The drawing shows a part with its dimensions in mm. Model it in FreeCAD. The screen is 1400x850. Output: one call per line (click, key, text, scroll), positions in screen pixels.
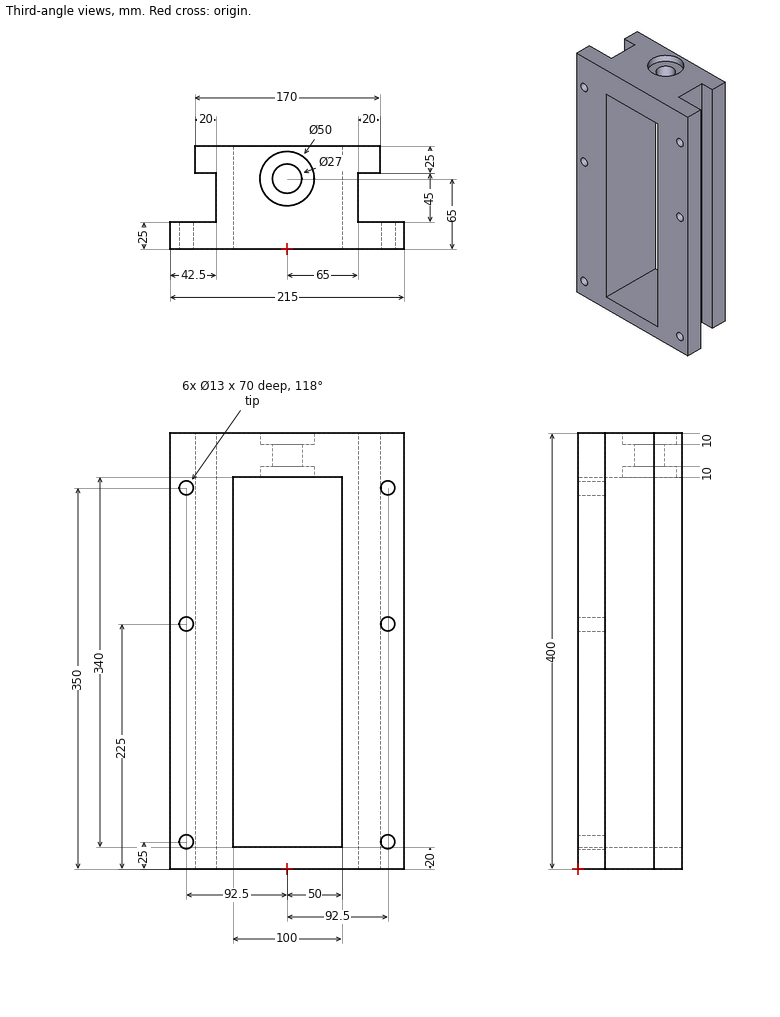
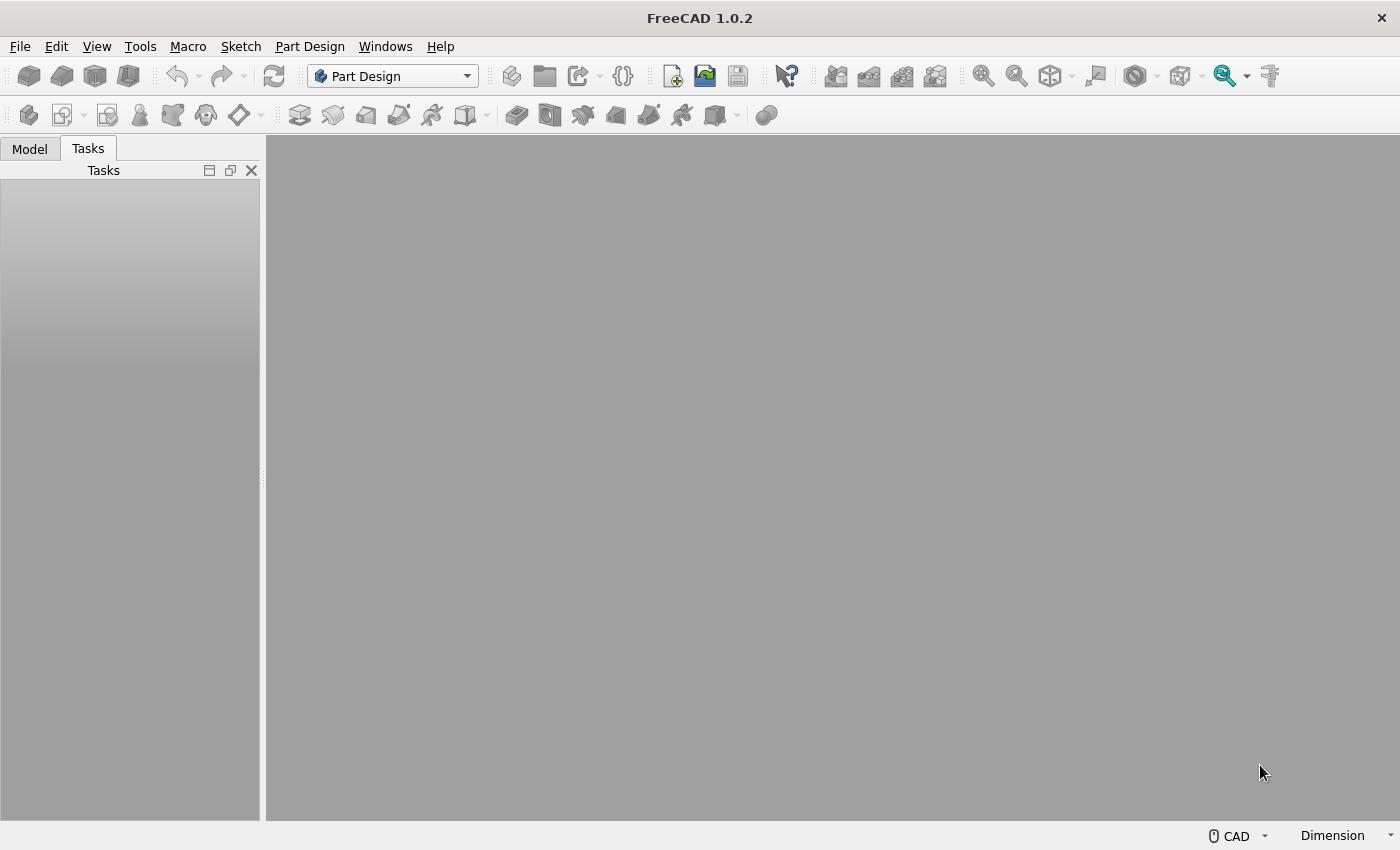
key(ctrl+n)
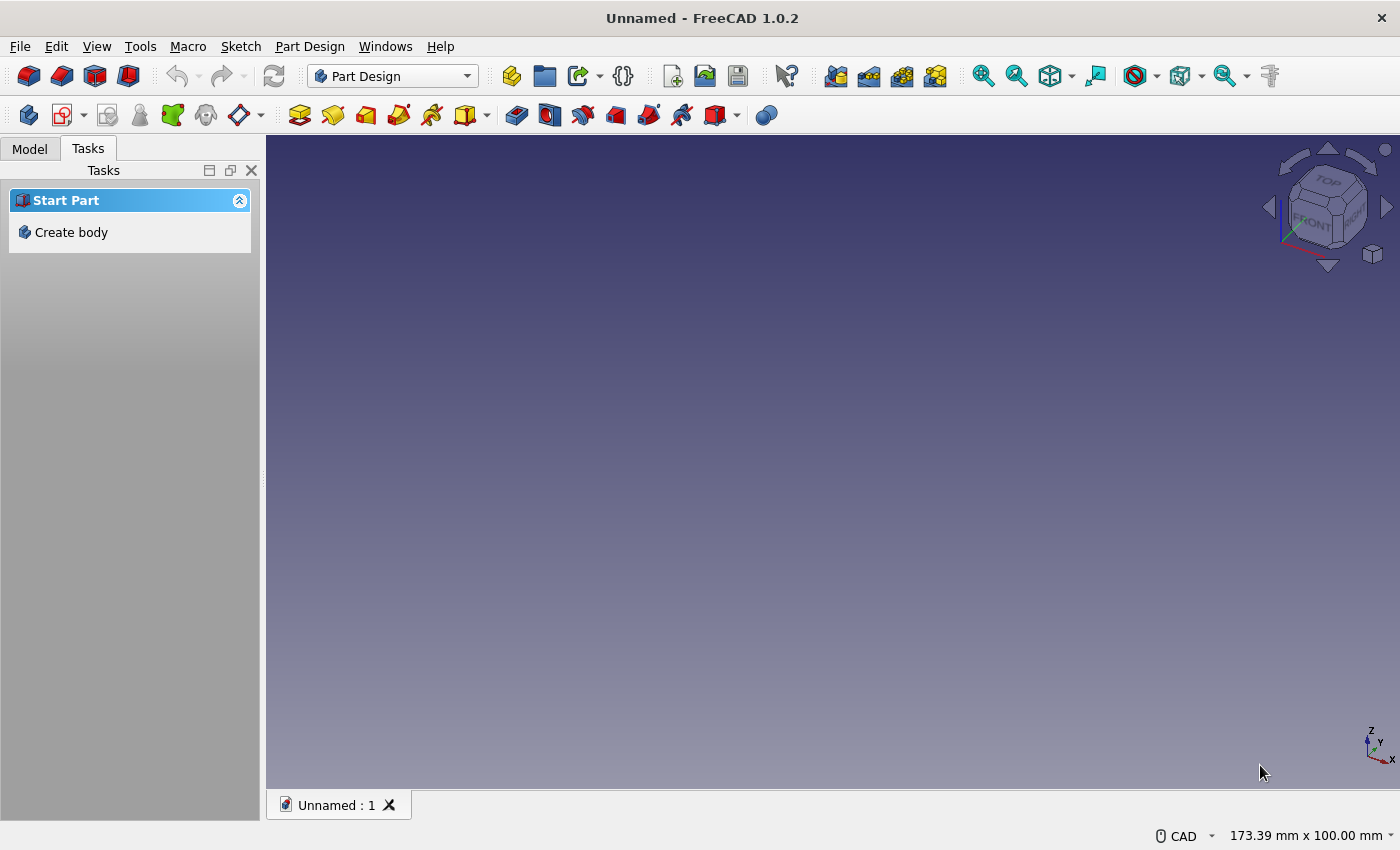
click(62, 116)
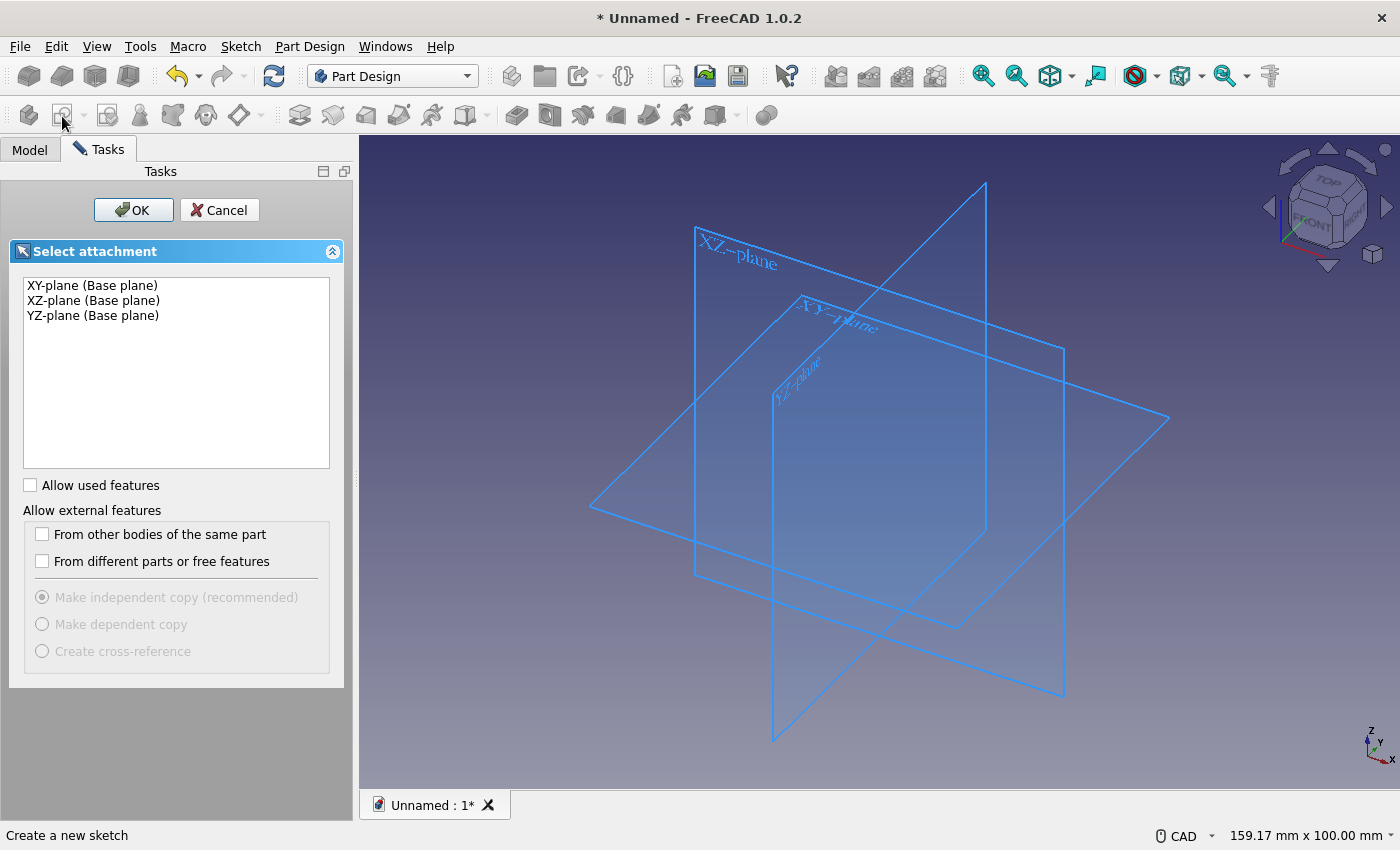
click(84, 286)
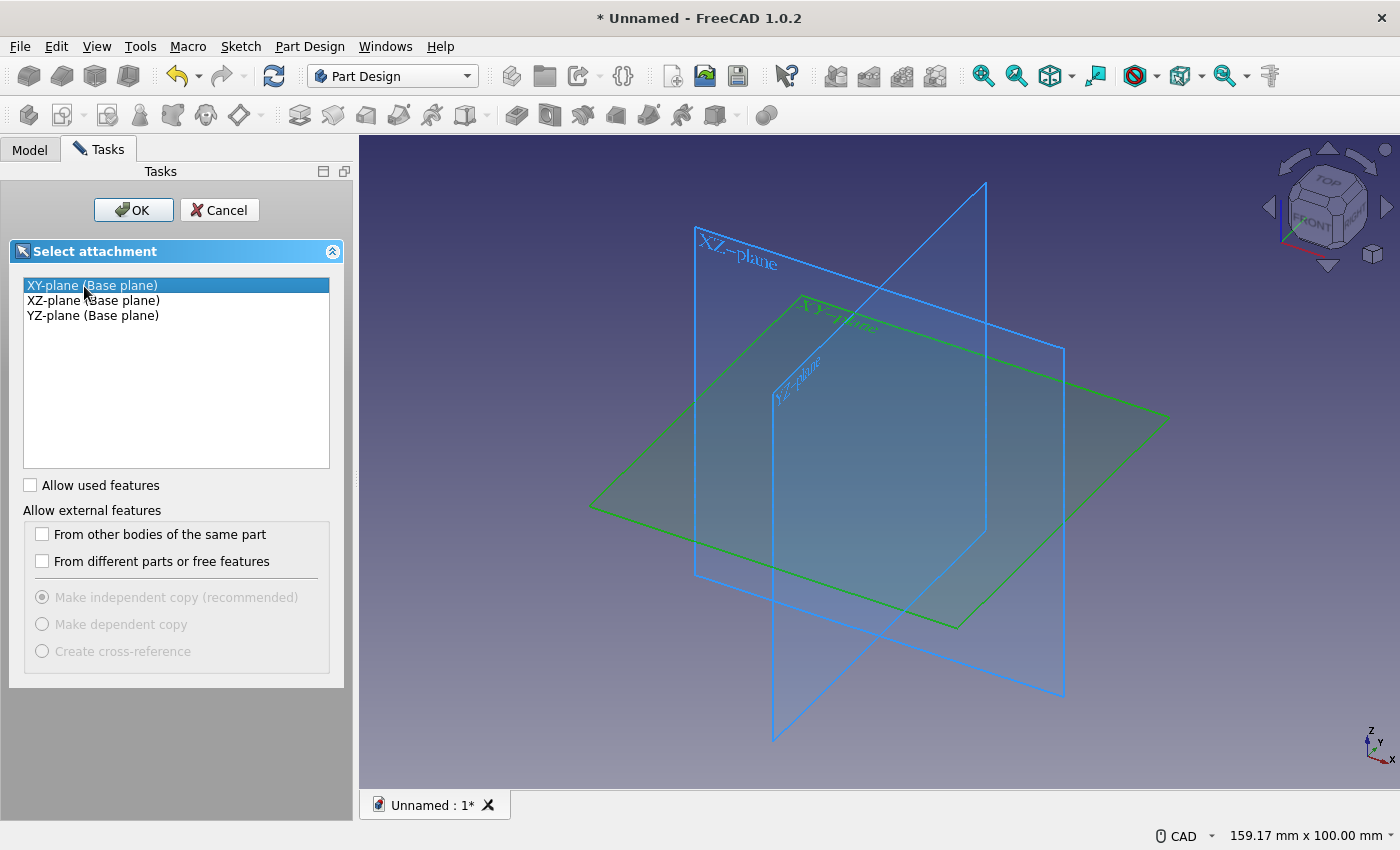
click(134, 210)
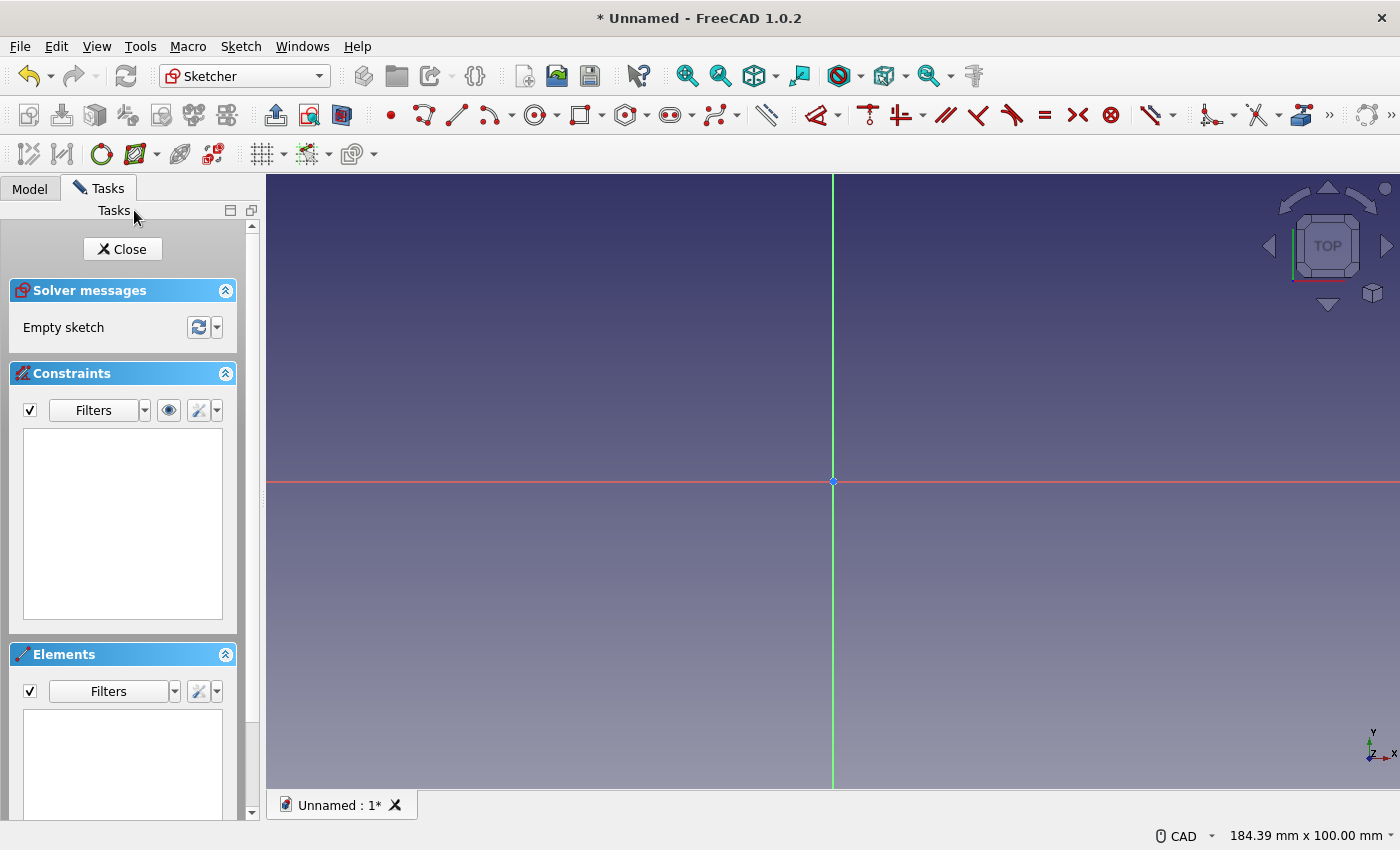
scroll(681, 761, down, 3)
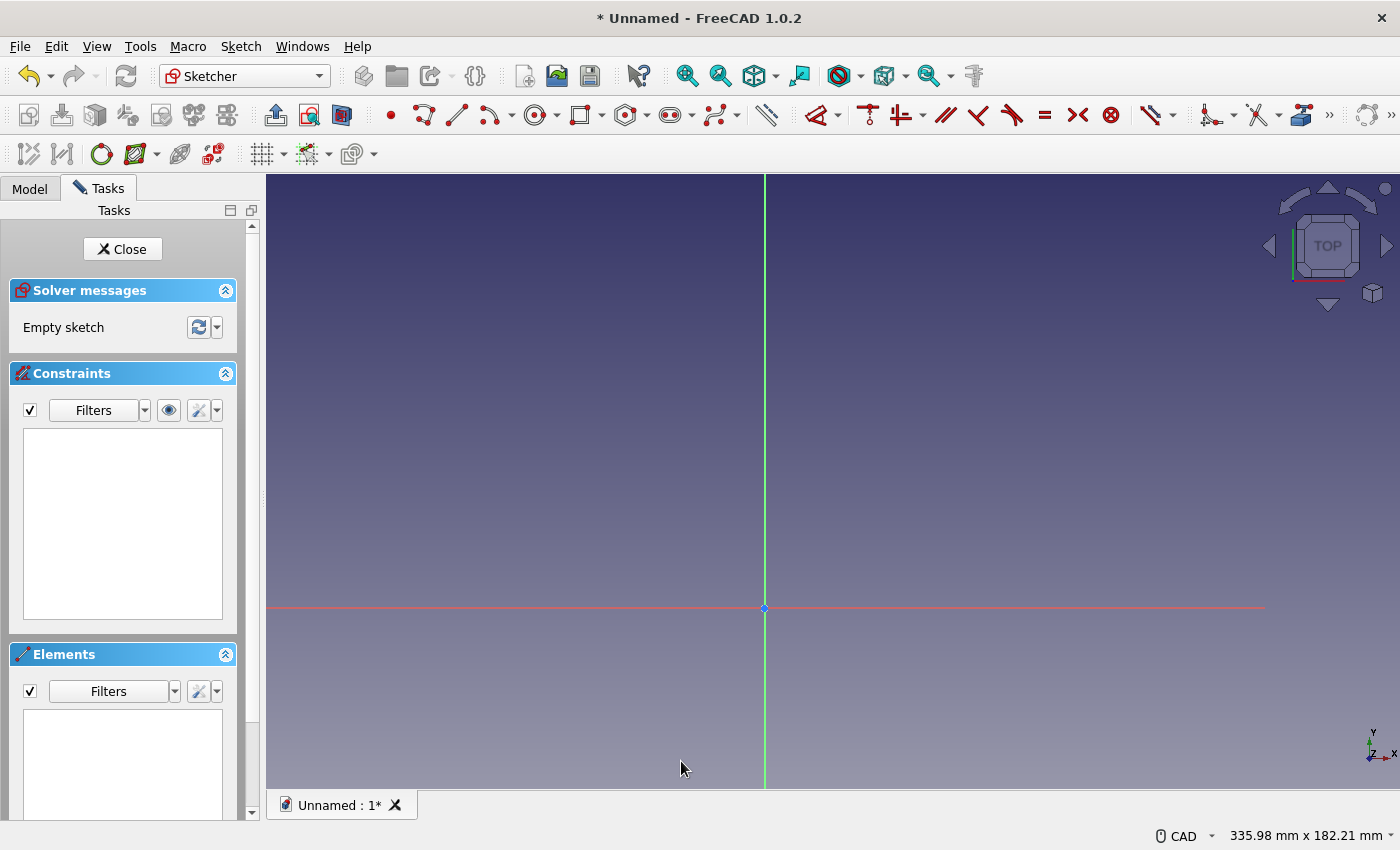
key(g)
key(m)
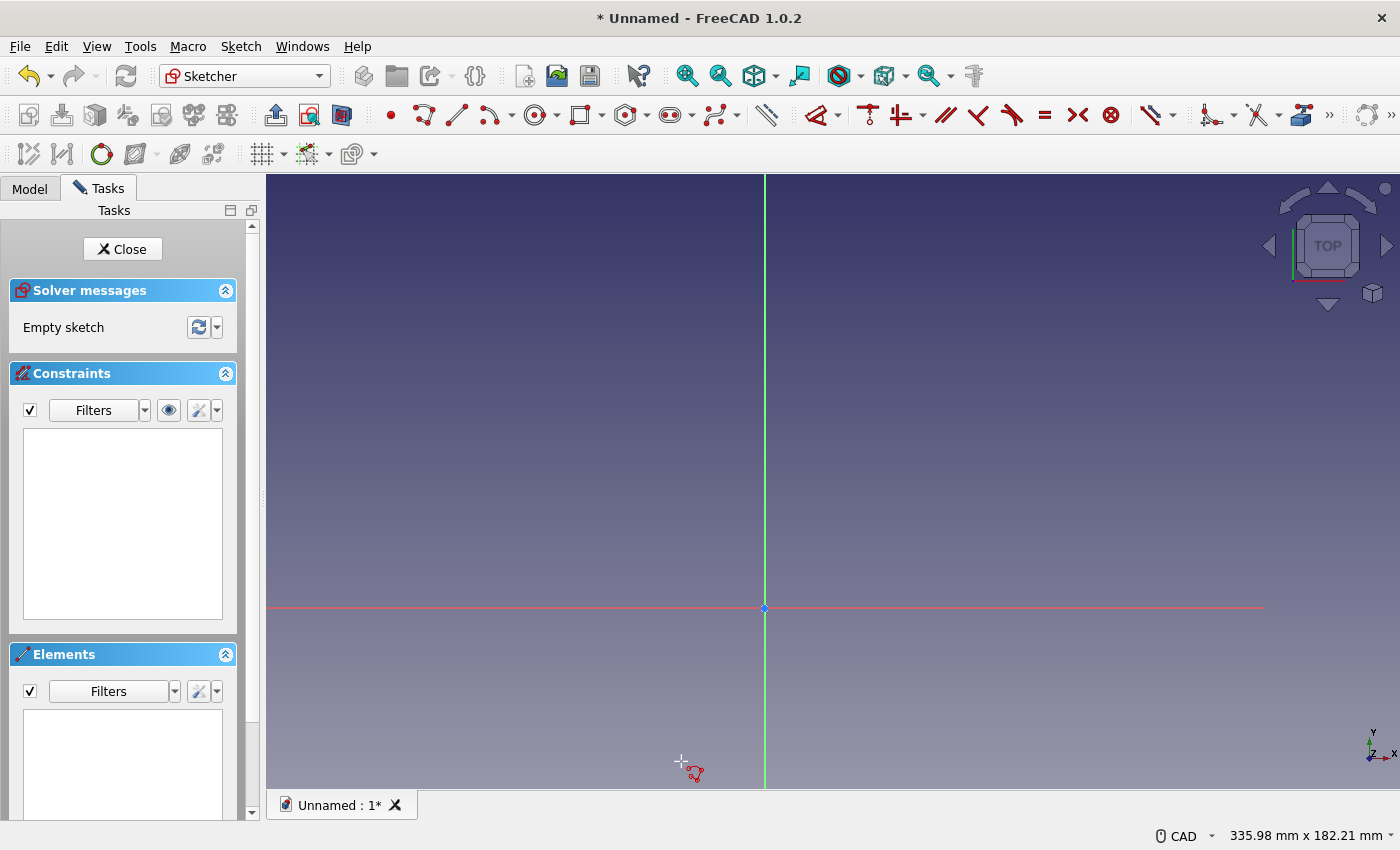
click(984, 524)
click(984, 372)
click(1051, 372)
click(1051, 287)
click(478, 287)
click(478, 372)
click(545, 372)
click(545, 524)
click(402, 524)
click(402, 608)
click(1127, 599)
click(1127, 524)
click(984, 525)
key(Escape)
key(Escape)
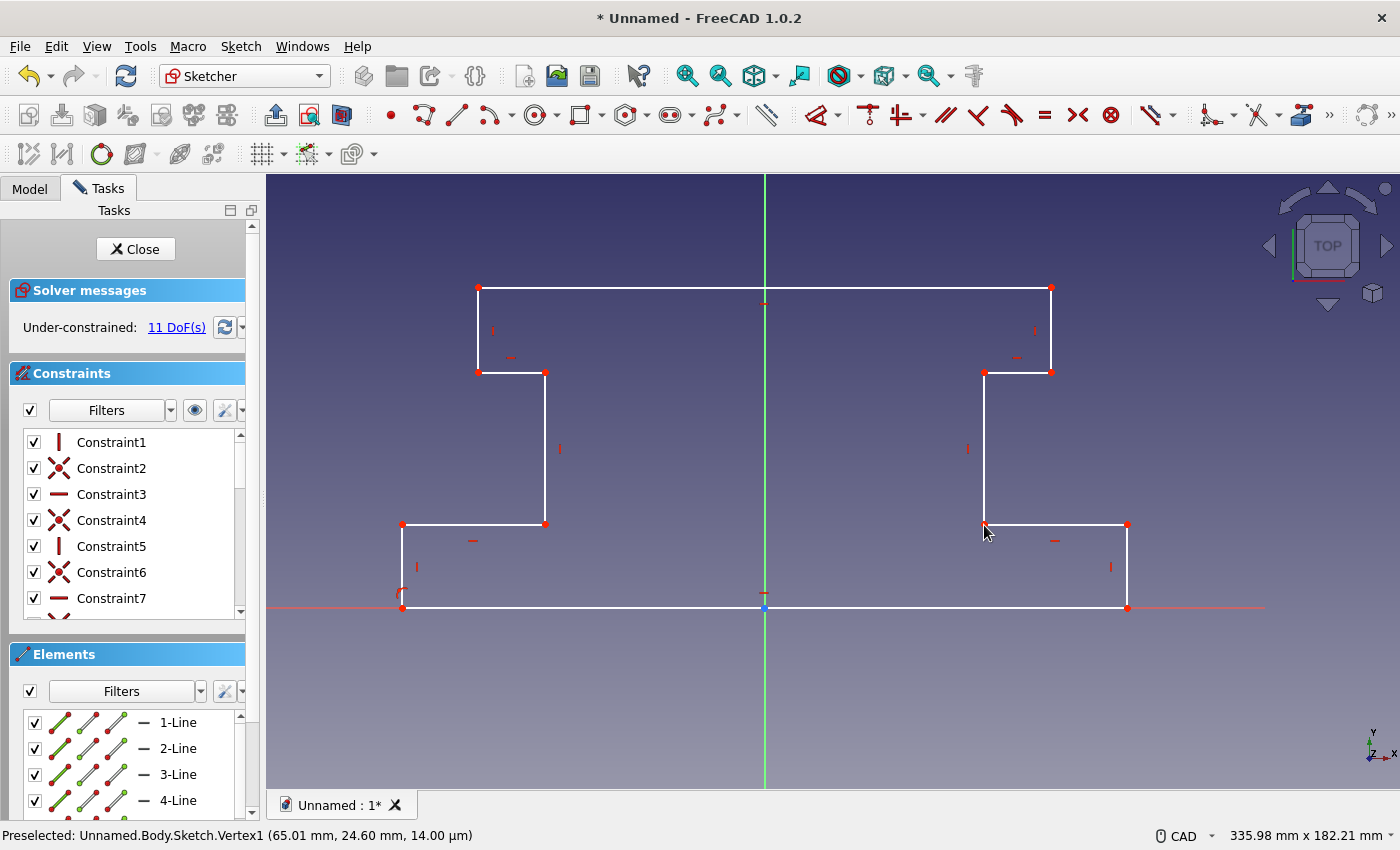
click(984, 479)